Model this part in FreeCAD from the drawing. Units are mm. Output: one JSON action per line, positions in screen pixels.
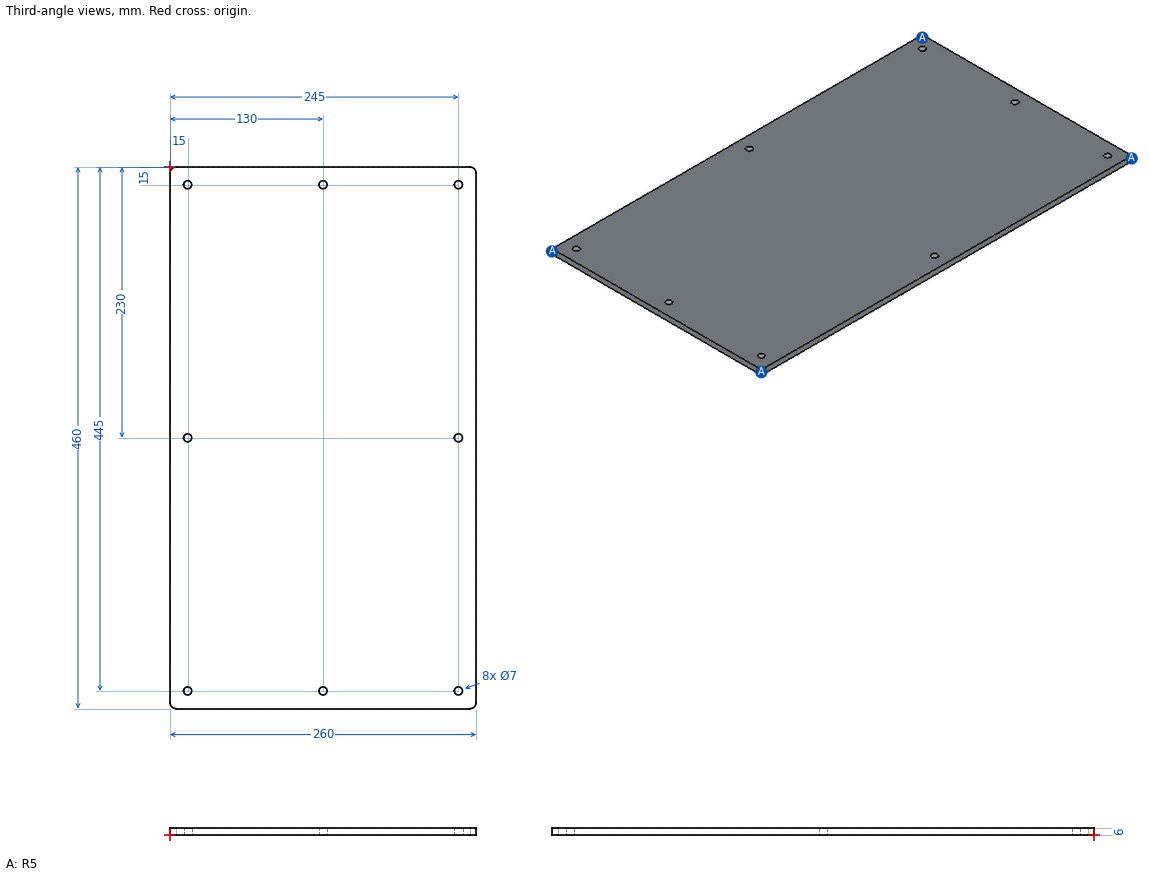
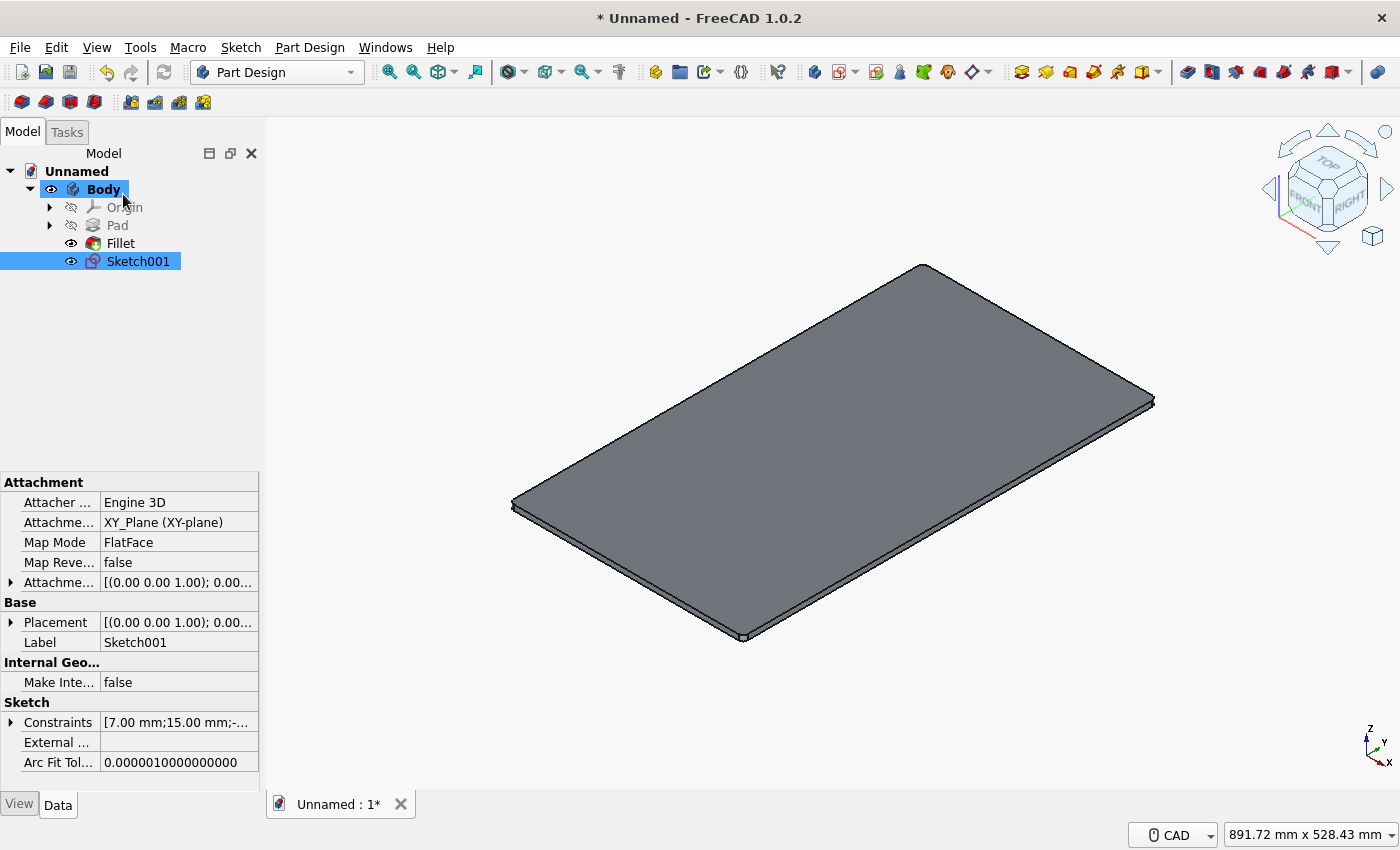
{"action": "left_click", "coordinate": [1188, 72]}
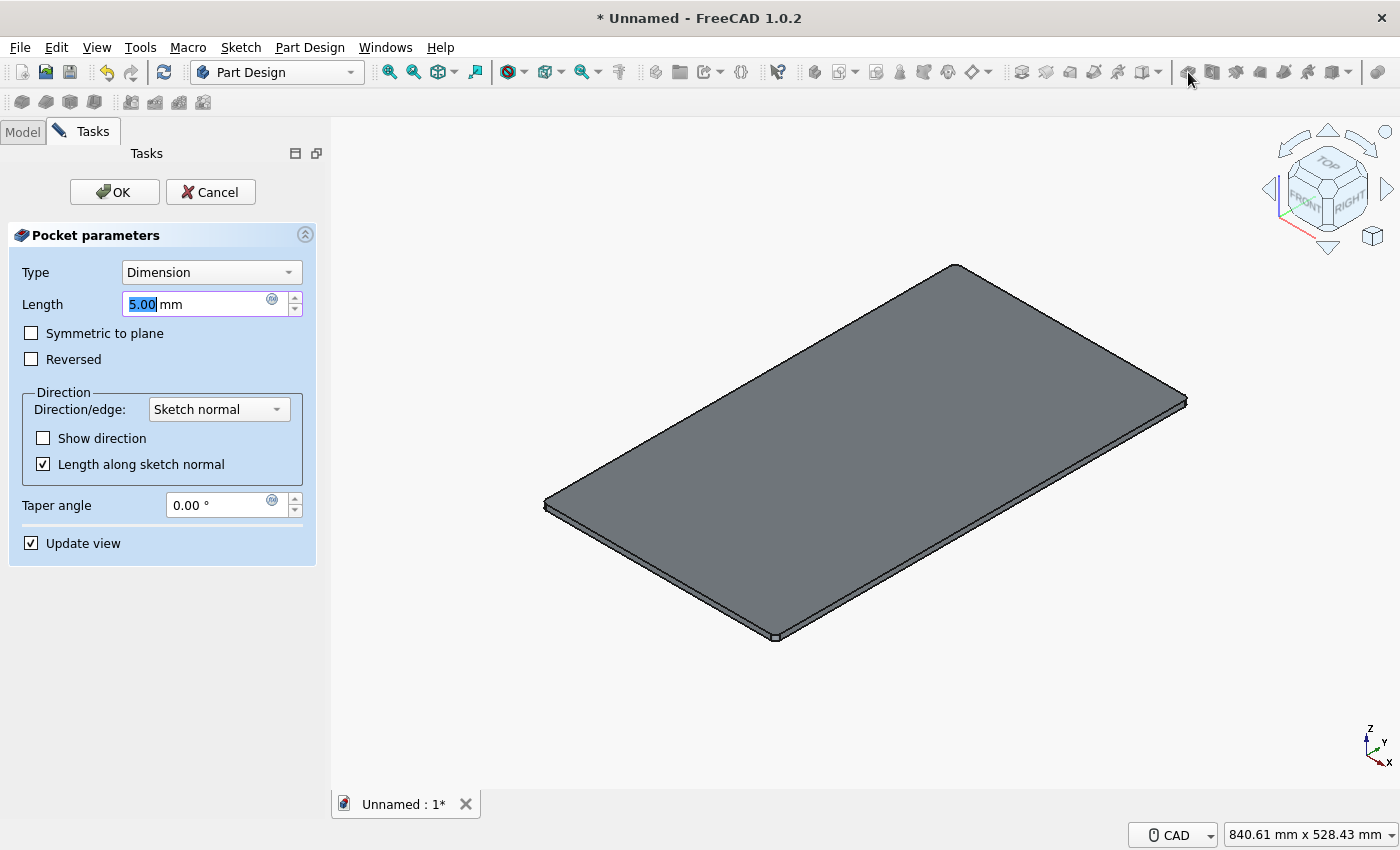
{"action": "left_click", "coordinate": [212, 272]}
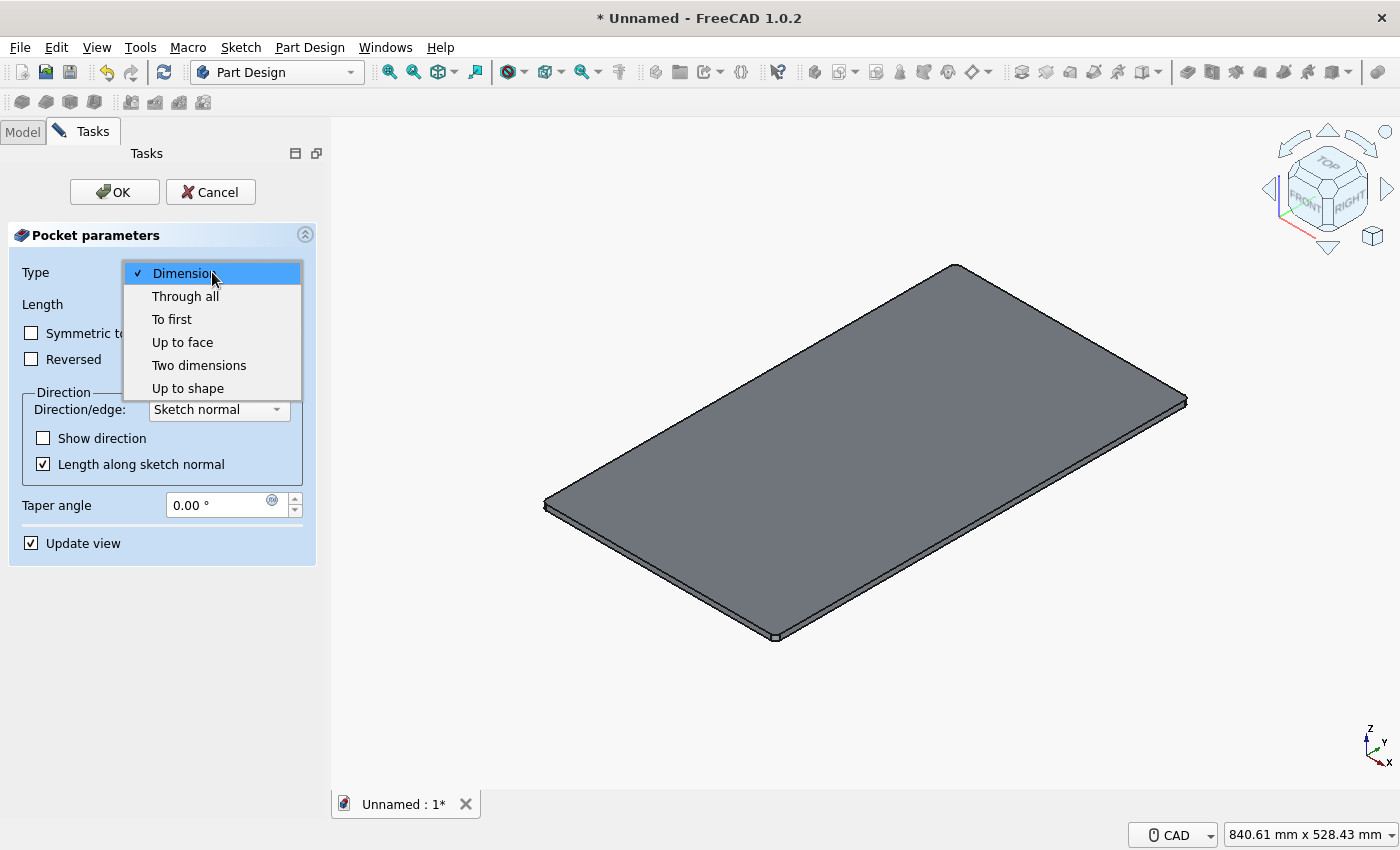
{"action": "left_click", "coordinate": [212, 296]}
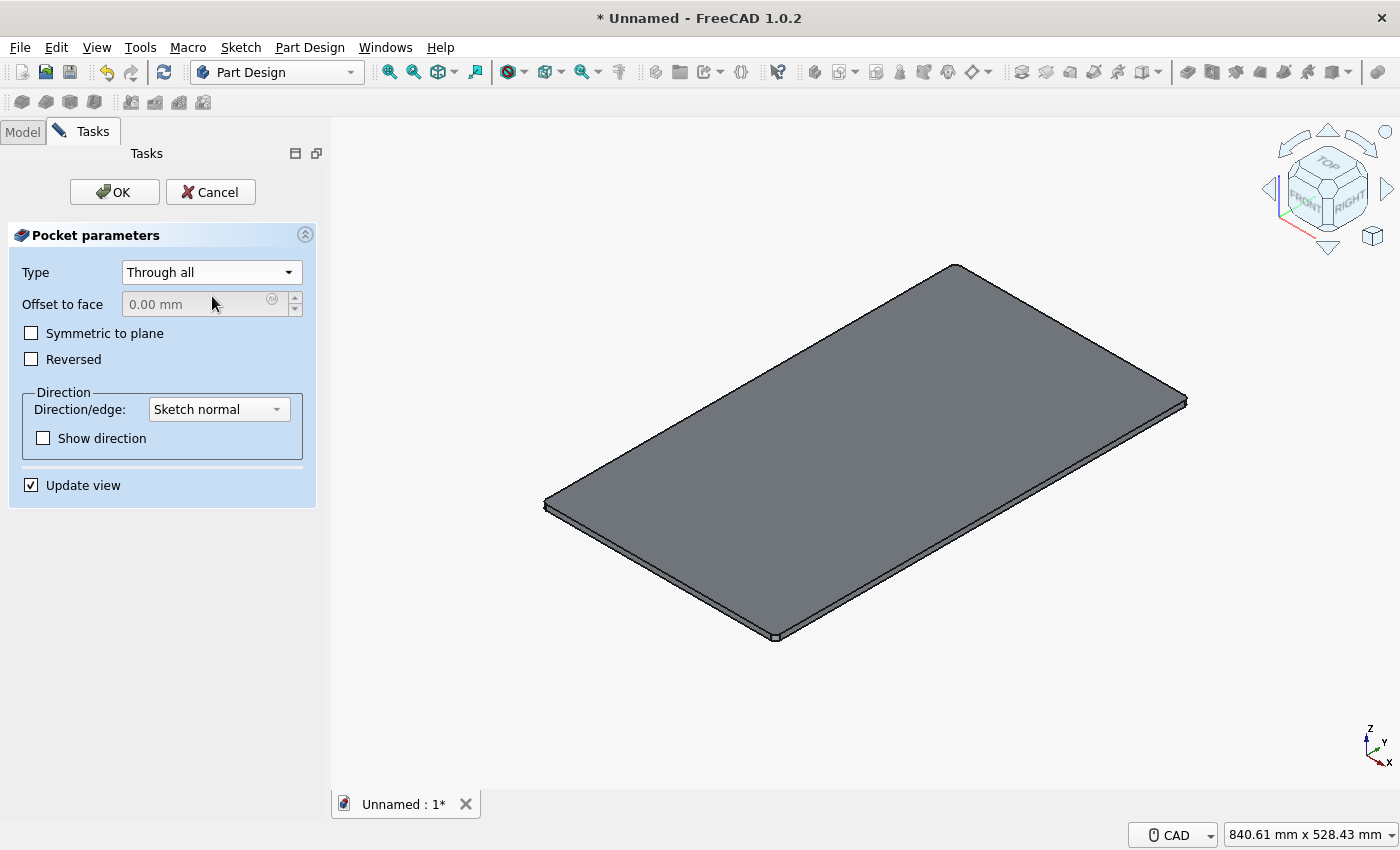
{"action": "left_click", "coordinate": [30, 359]}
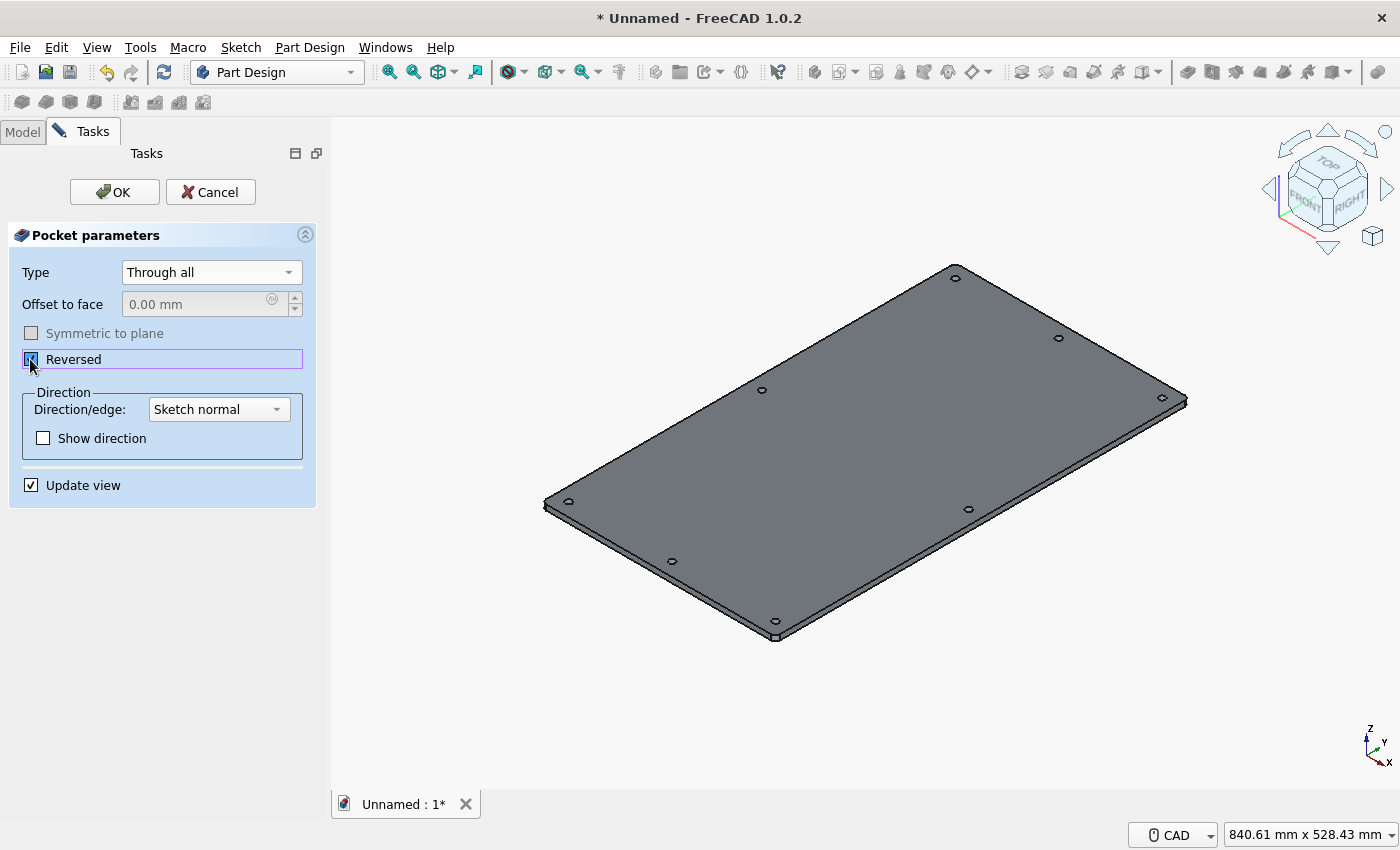
{"action": "left_click", "coordinate": [115, 192]}